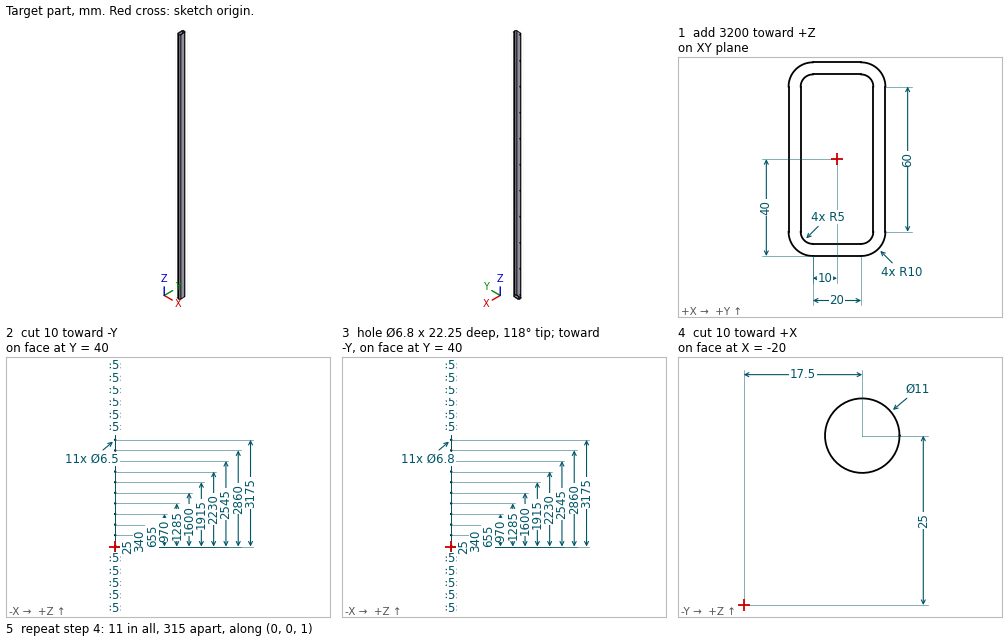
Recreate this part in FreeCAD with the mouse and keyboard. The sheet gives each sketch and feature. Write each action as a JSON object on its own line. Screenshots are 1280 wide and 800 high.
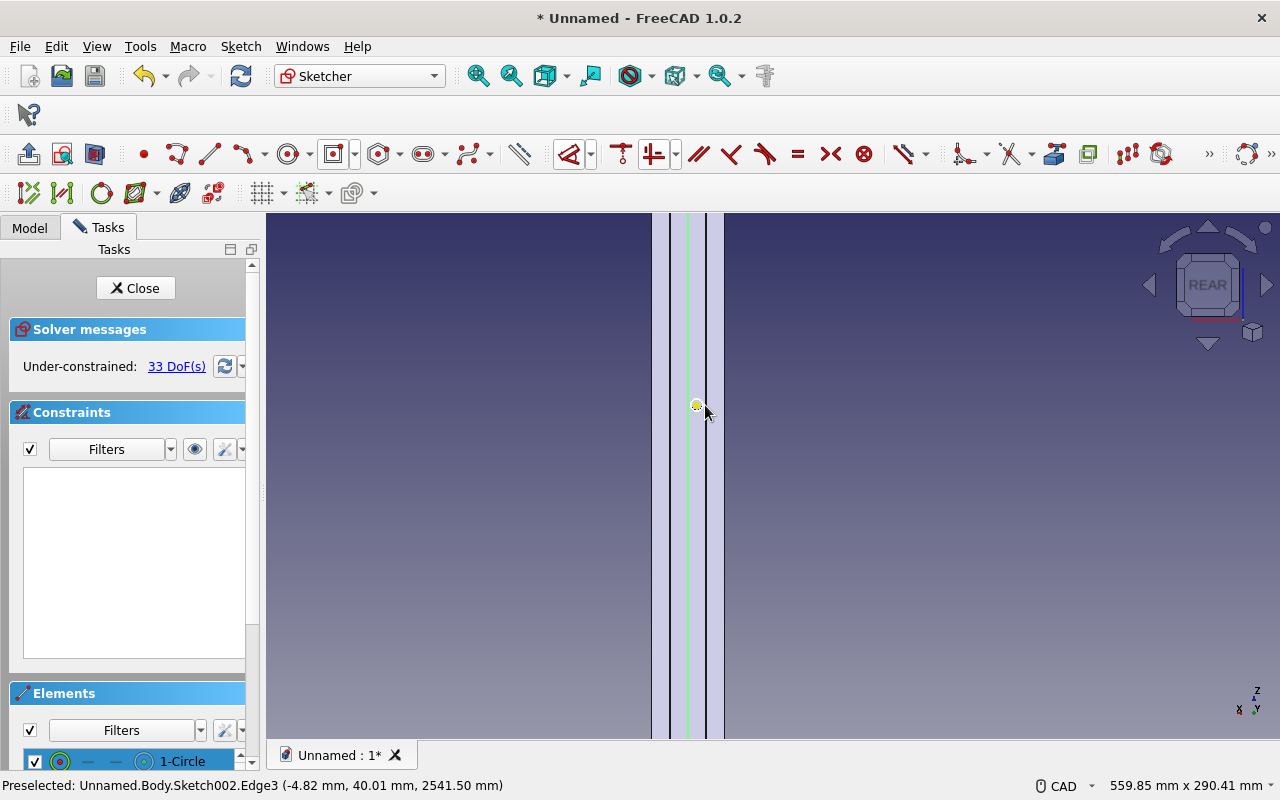
{"action": "left_click", "coordinate": [691, 405]}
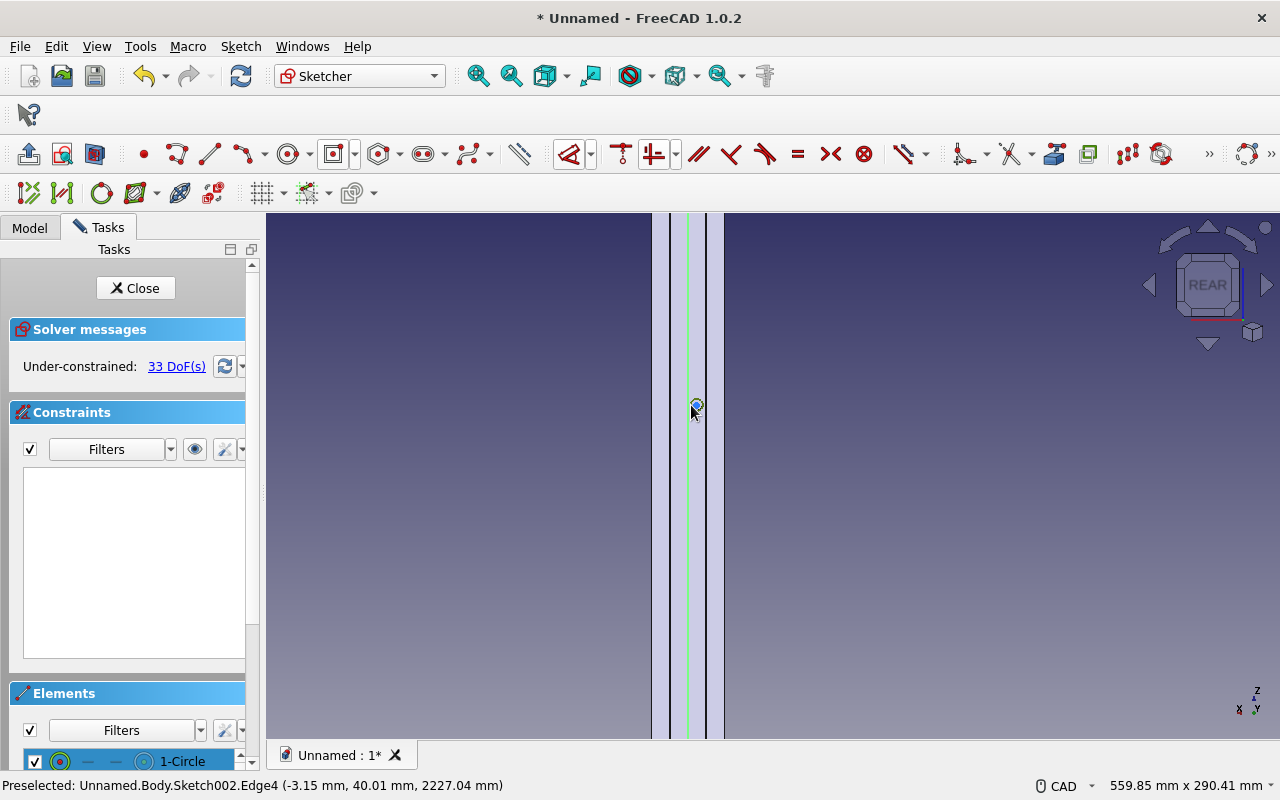
{"action": "scroll", "coordinate": [705, 405], "scroll_direction": "down", "scroll_amount": 14}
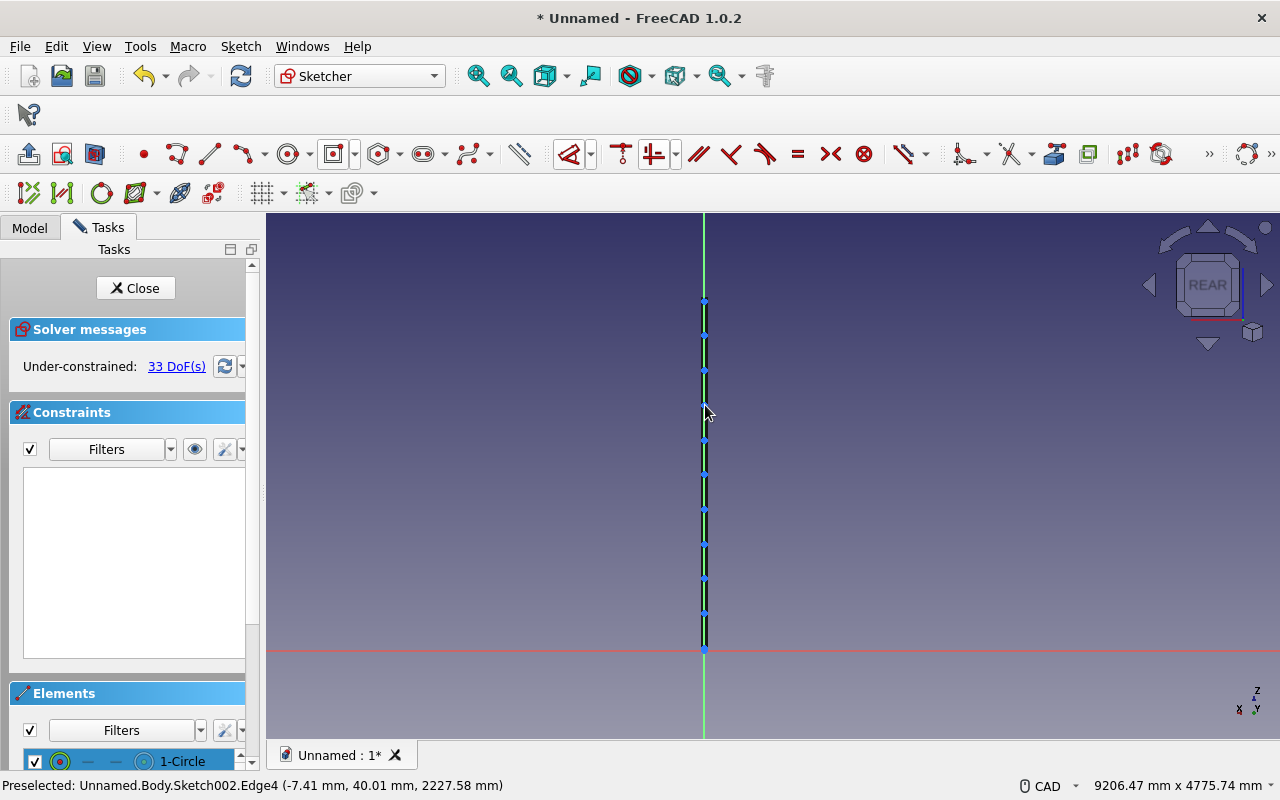
{"action": "scroll", "coordinate": [705, 440], "scroll_direction": "up", "scroll_amount": 14}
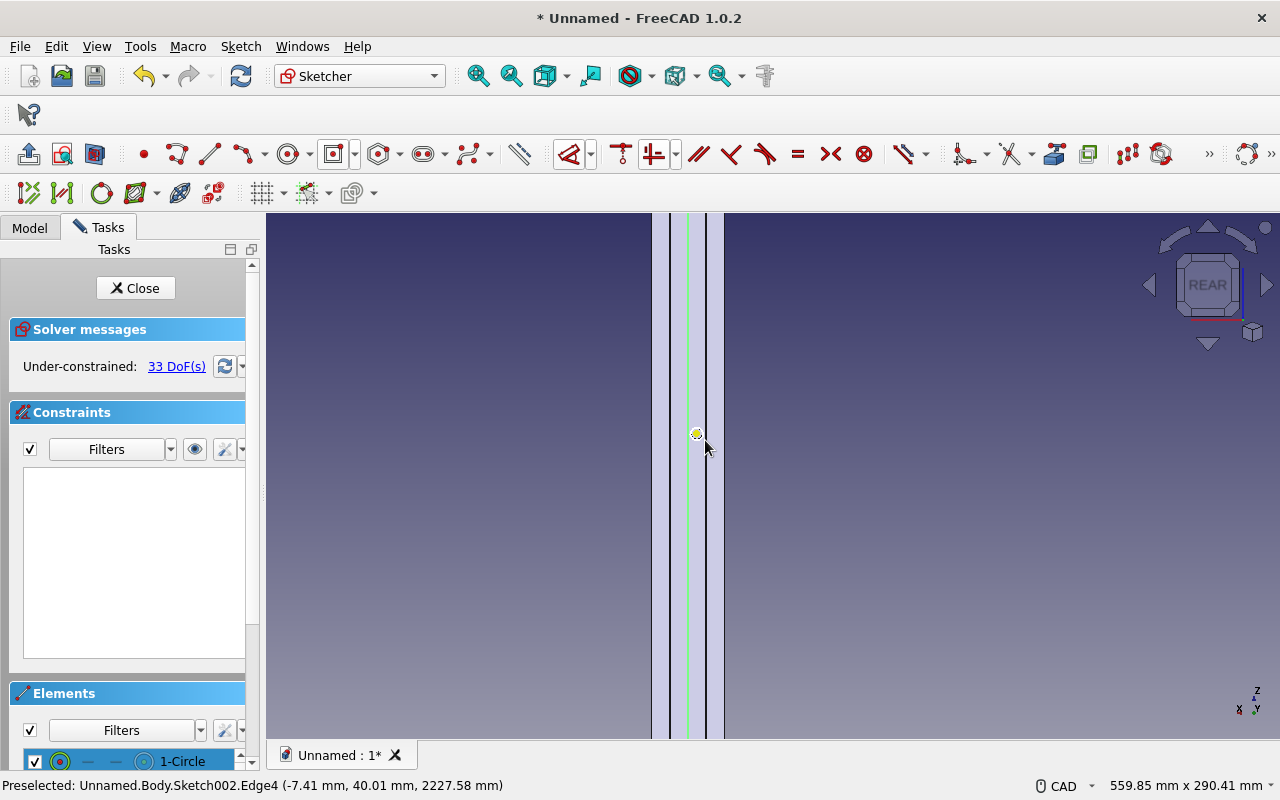
{"action": "left_click", "coordinate": [697, 428]}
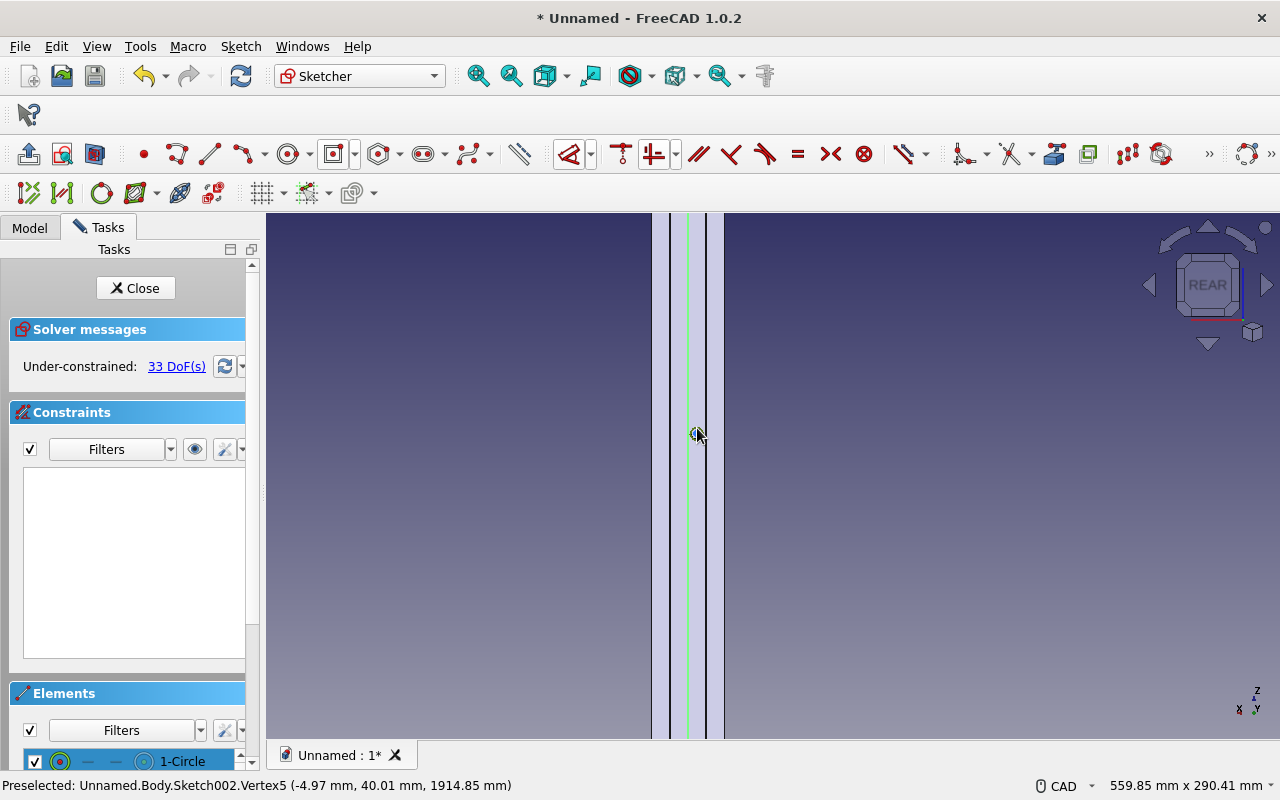
{"action": "scroll", "coordinate": [705, 441], "scroll_direction": "down", "scroll_amount": 14}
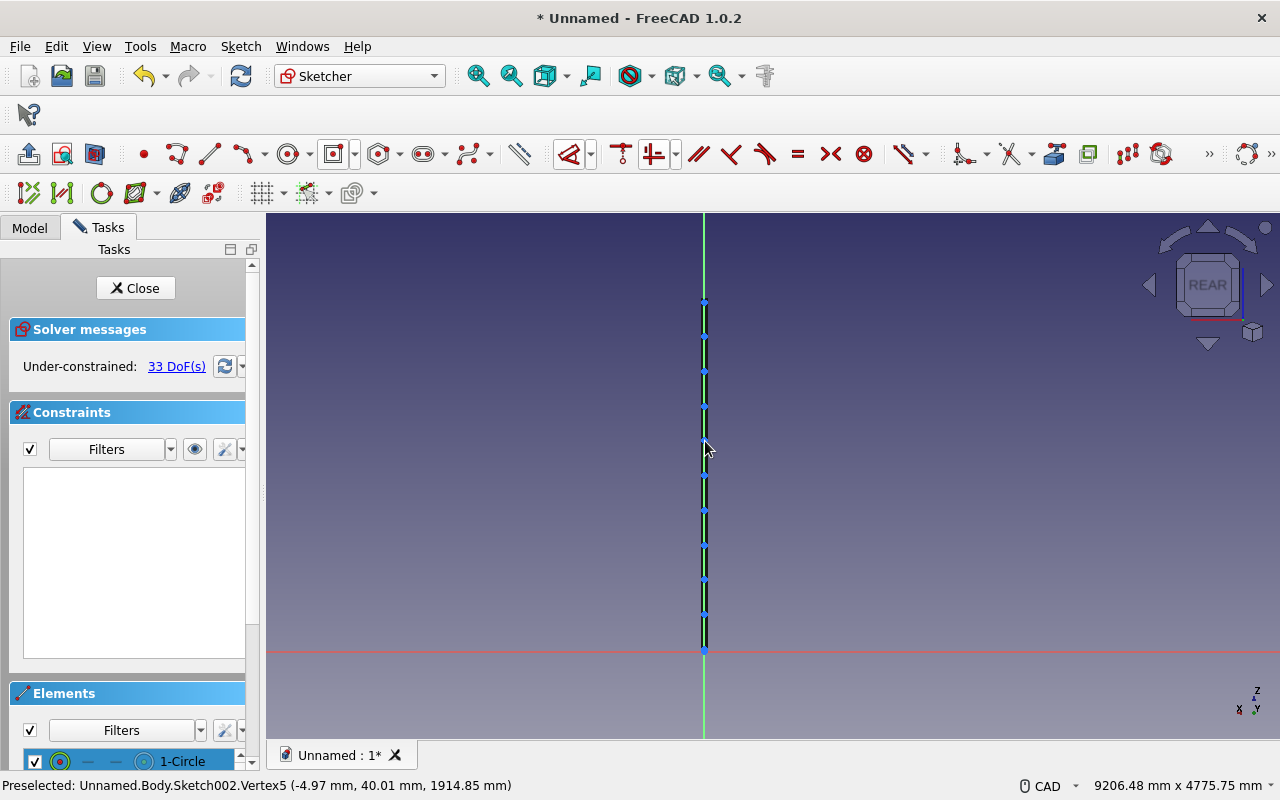
{"action": "scroll", "coordinate": [705, 475], "scroll_direction": "up", "scroll_amount": 14}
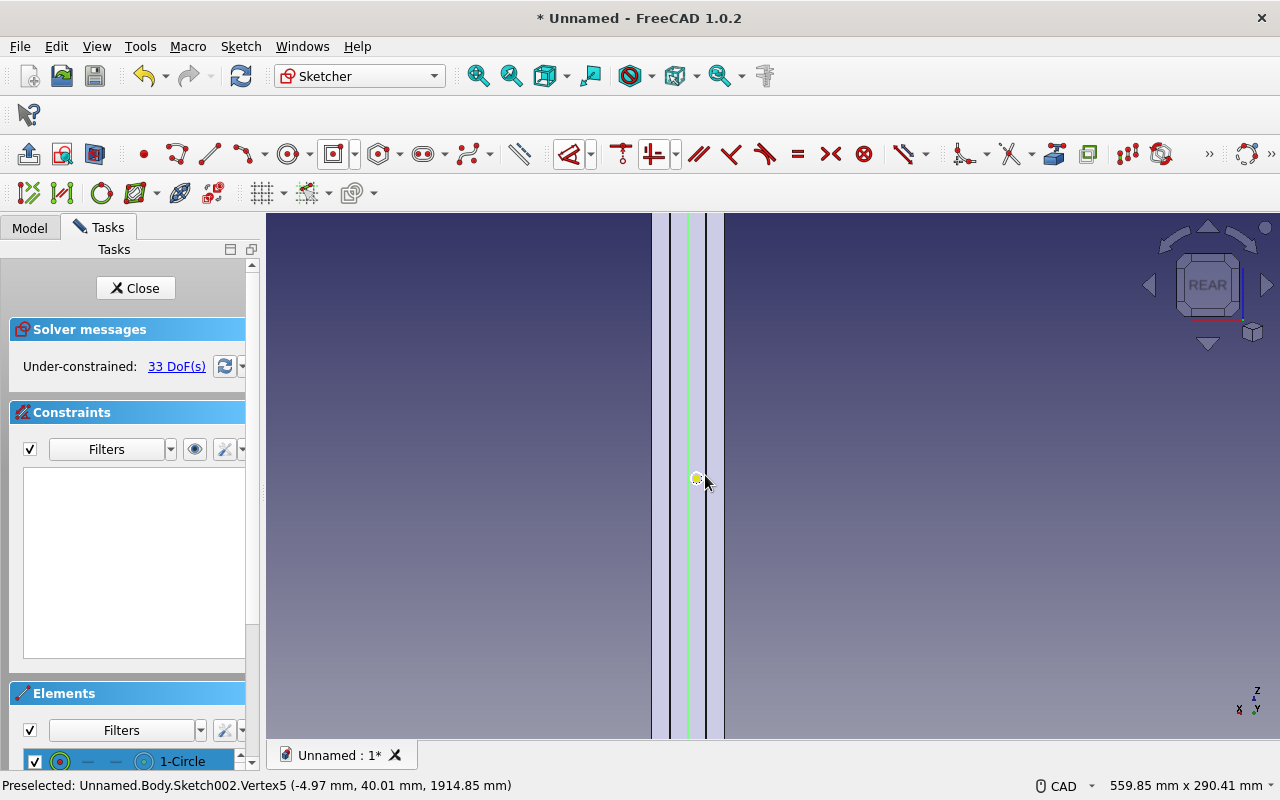
{"action": "left_click", "coordinate": [701, 474]}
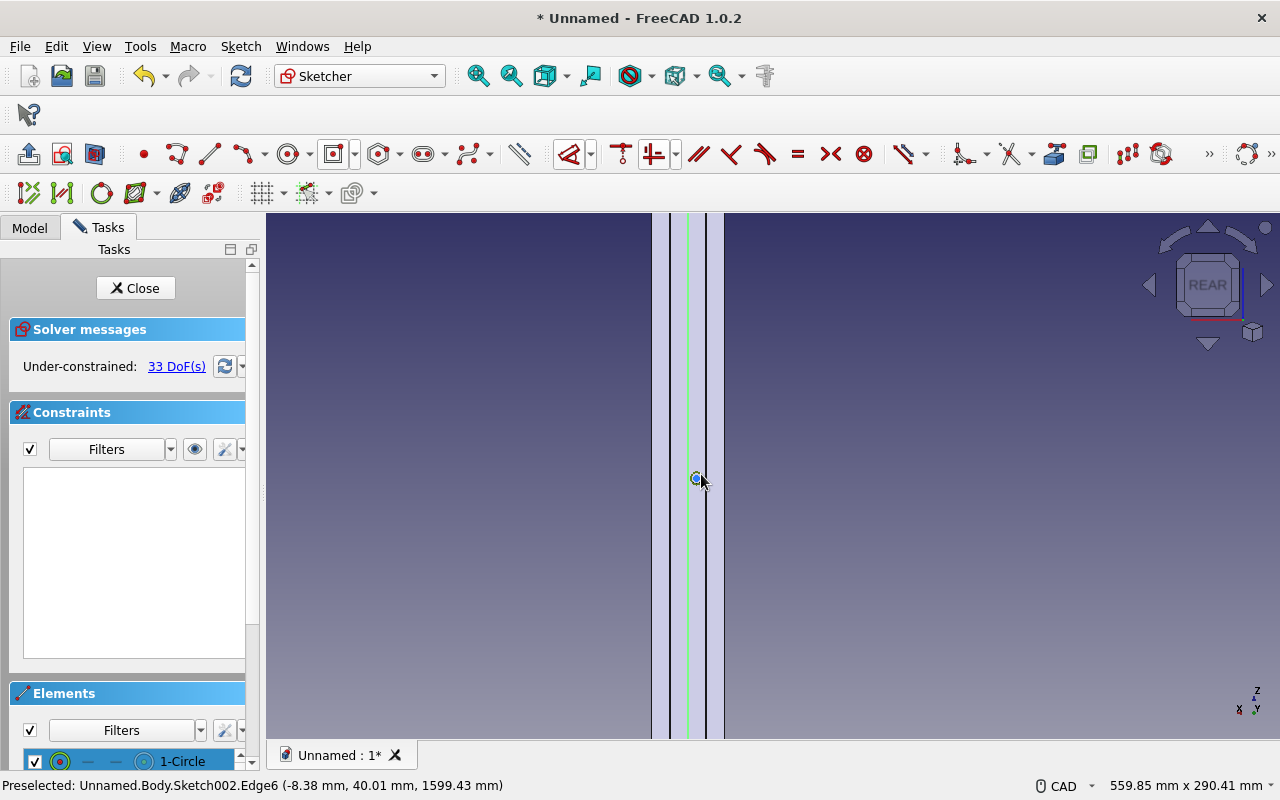
{"action": "scroll", "coordinate": [705, 475], "scroll_direction": "down", "scroll_amount": 14}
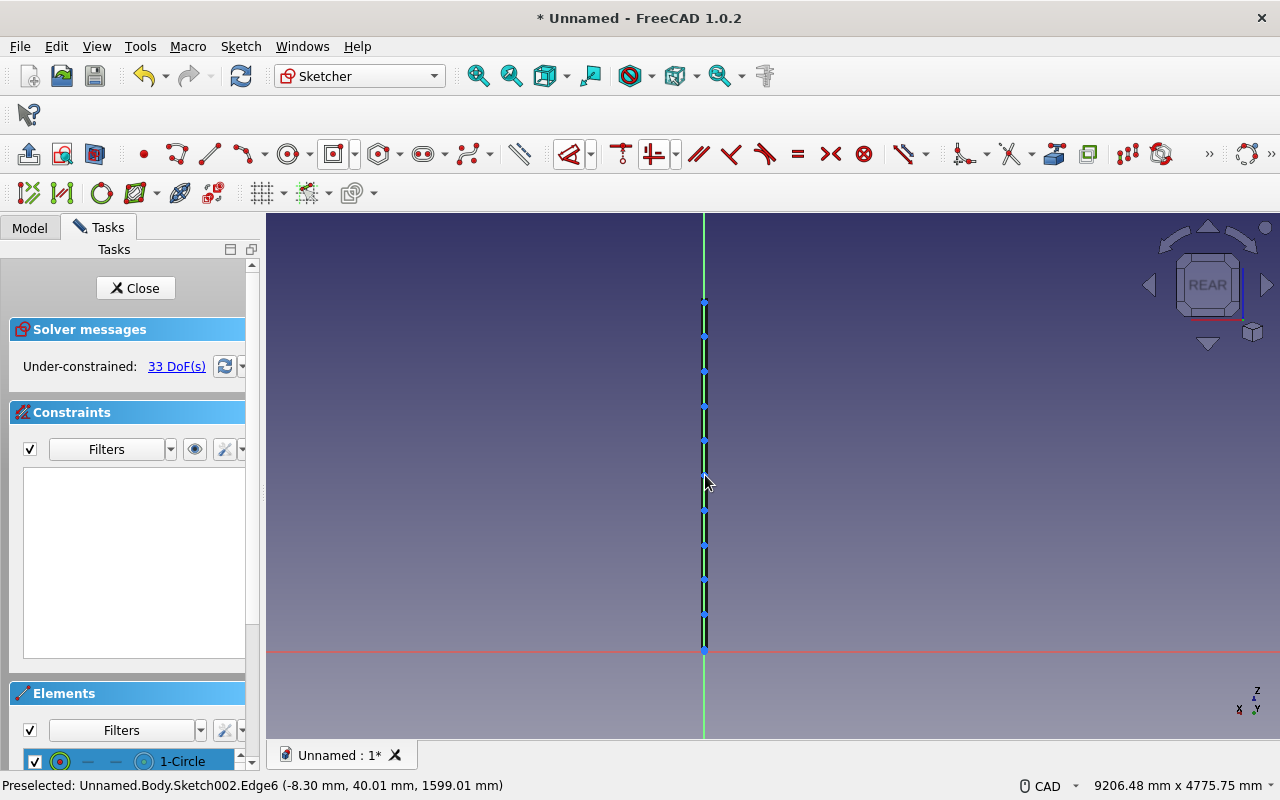
{"action": "scroll", "coordinate": [705, 510], "scroll_direction": "up", "scroll_amount": 14}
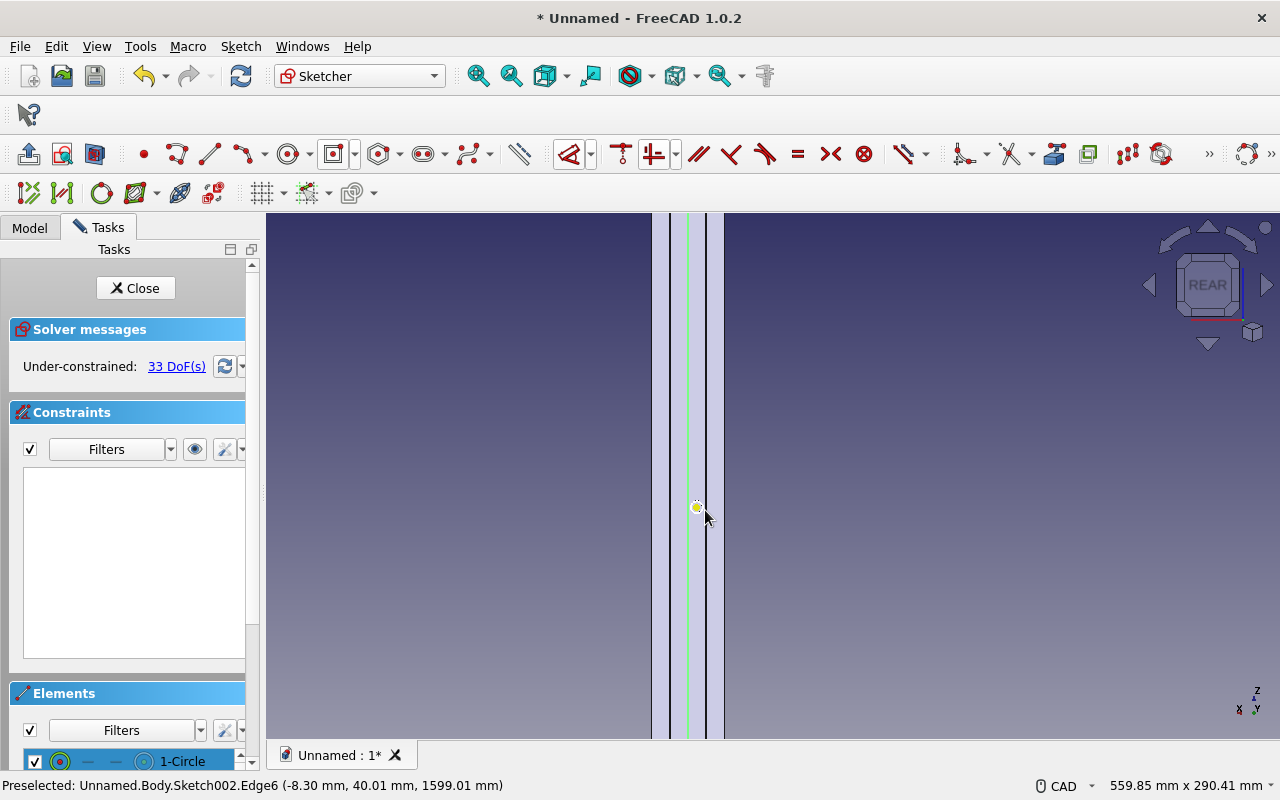
{"action": "left_click", "coordinate": [697, 501]}